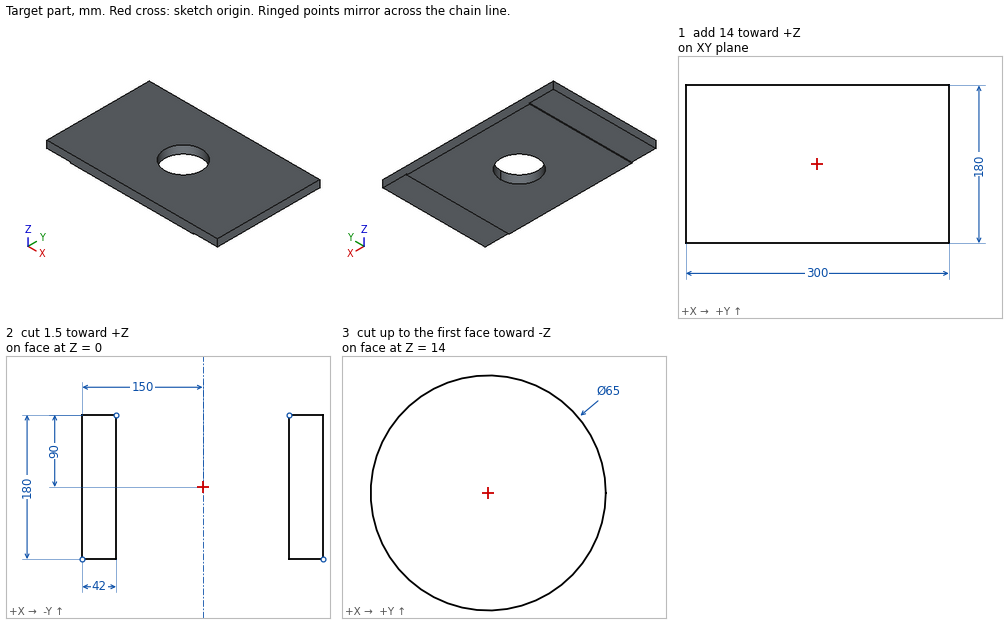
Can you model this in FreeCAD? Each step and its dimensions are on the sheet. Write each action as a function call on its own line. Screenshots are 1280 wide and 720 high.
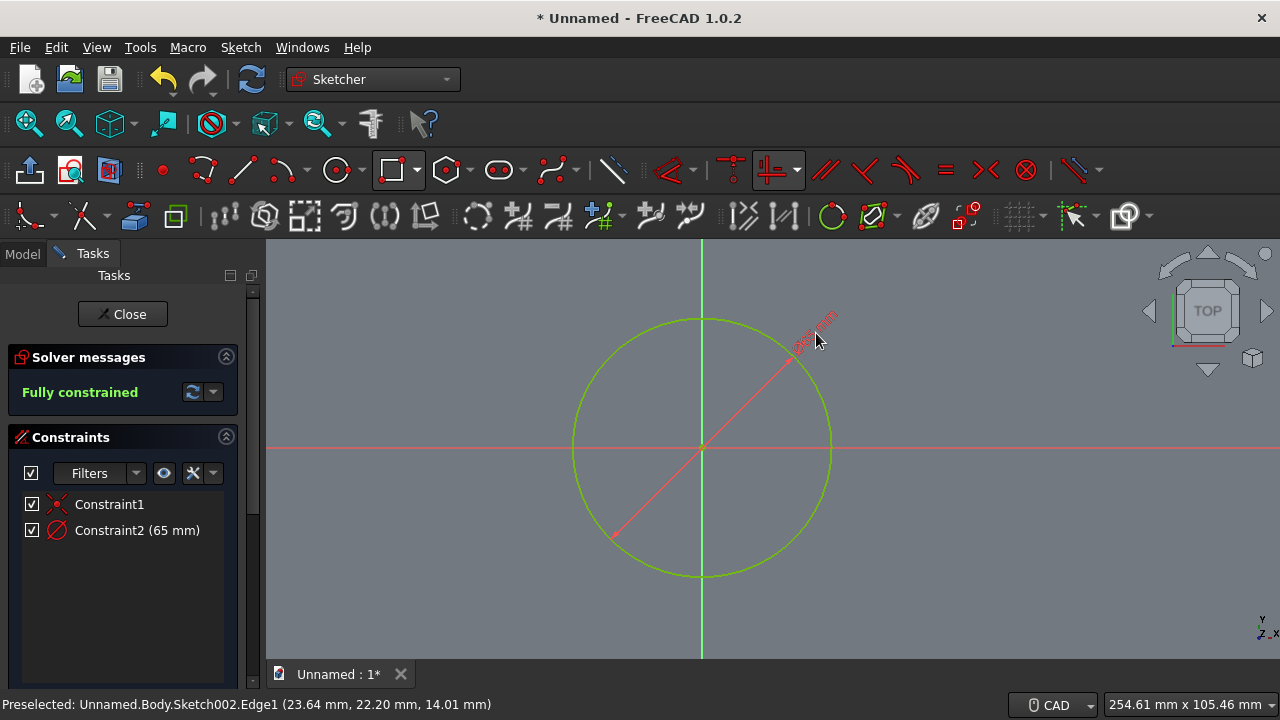
click(123, 314)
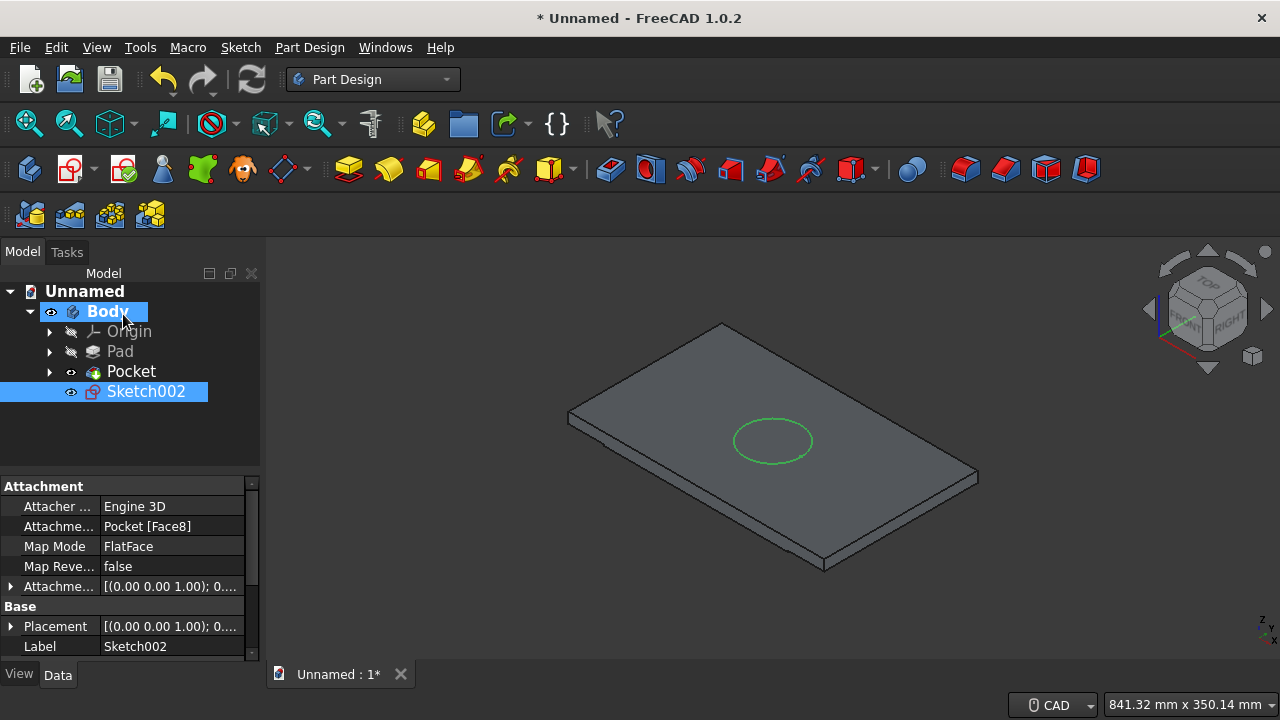
click(612, 170)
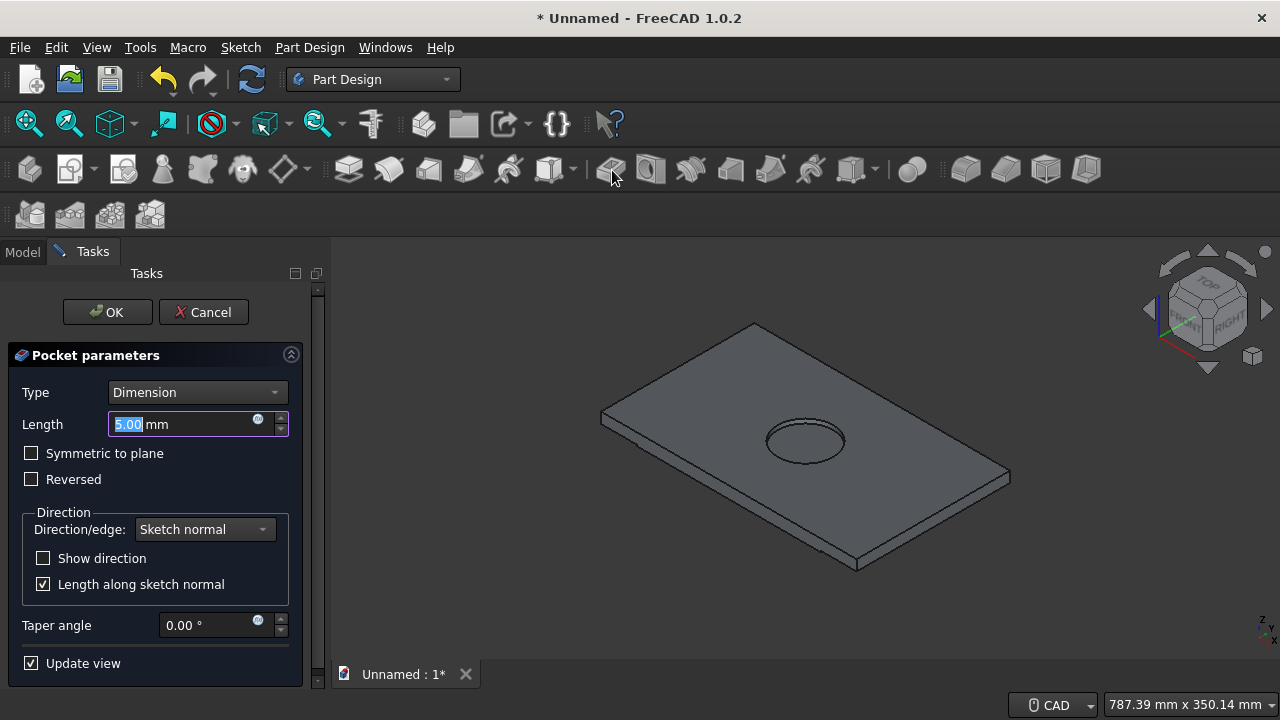
click(198, 392)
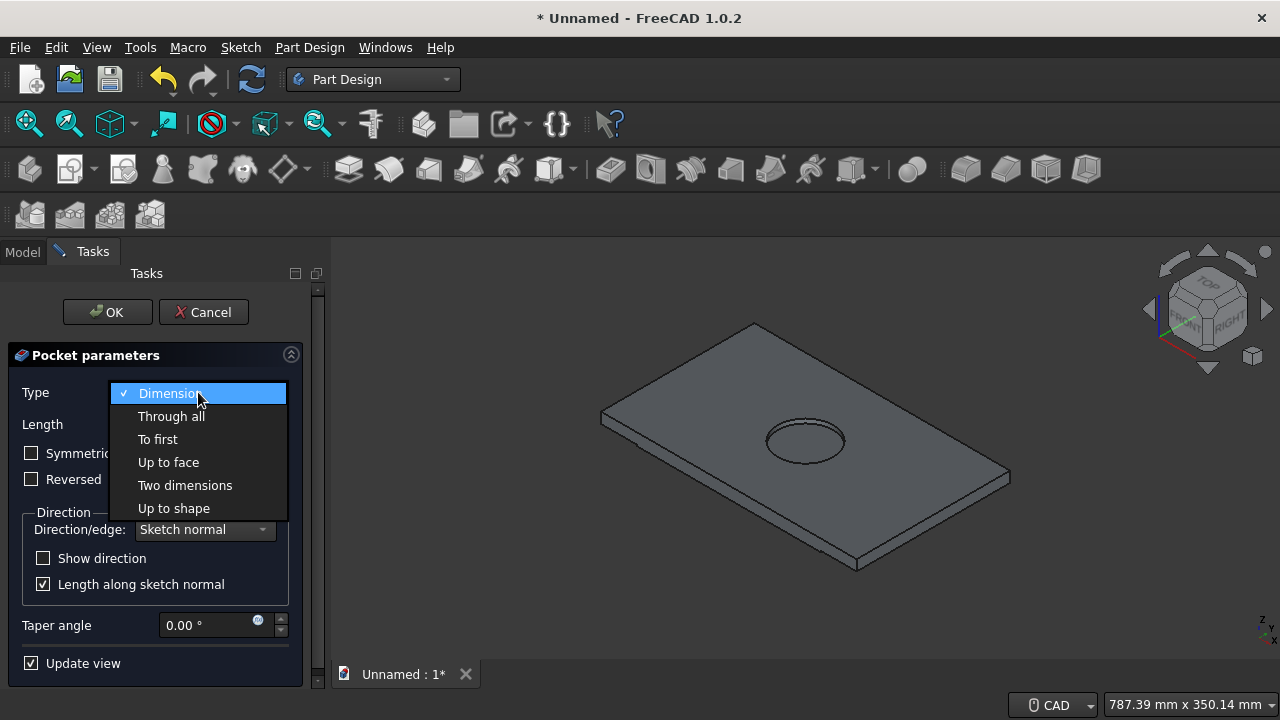
click(198, 440)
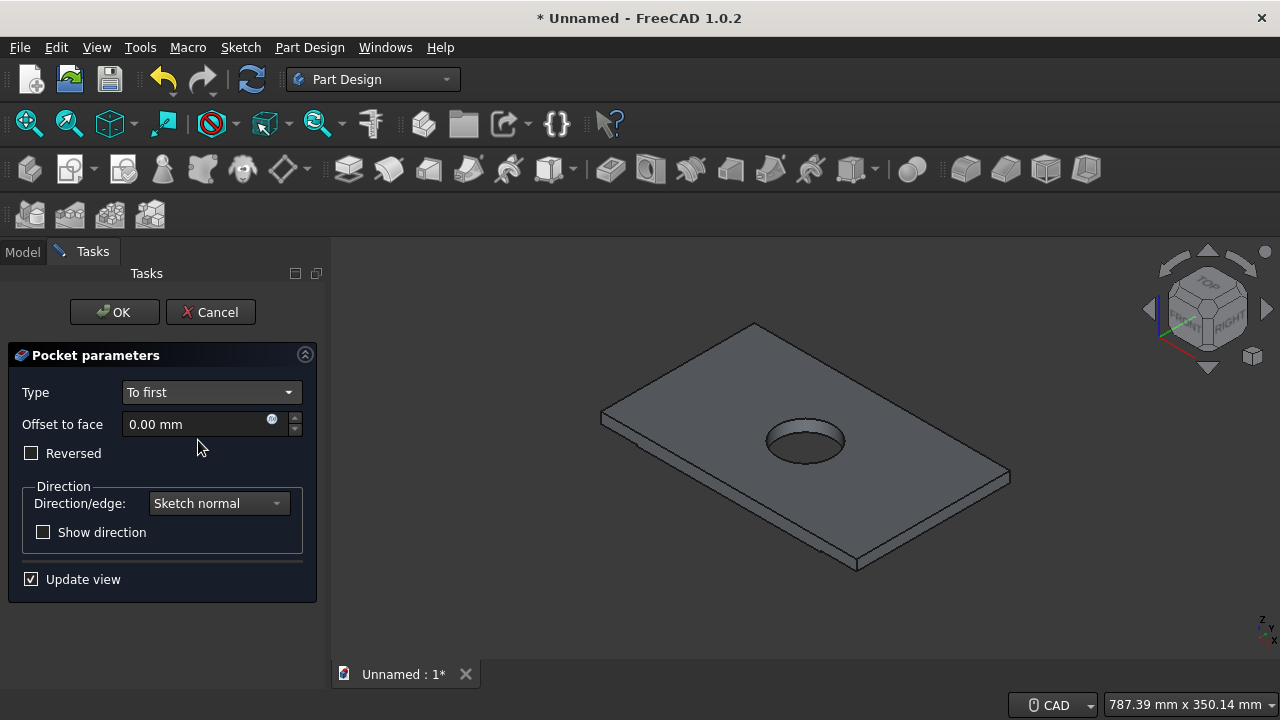
click(115, 312)